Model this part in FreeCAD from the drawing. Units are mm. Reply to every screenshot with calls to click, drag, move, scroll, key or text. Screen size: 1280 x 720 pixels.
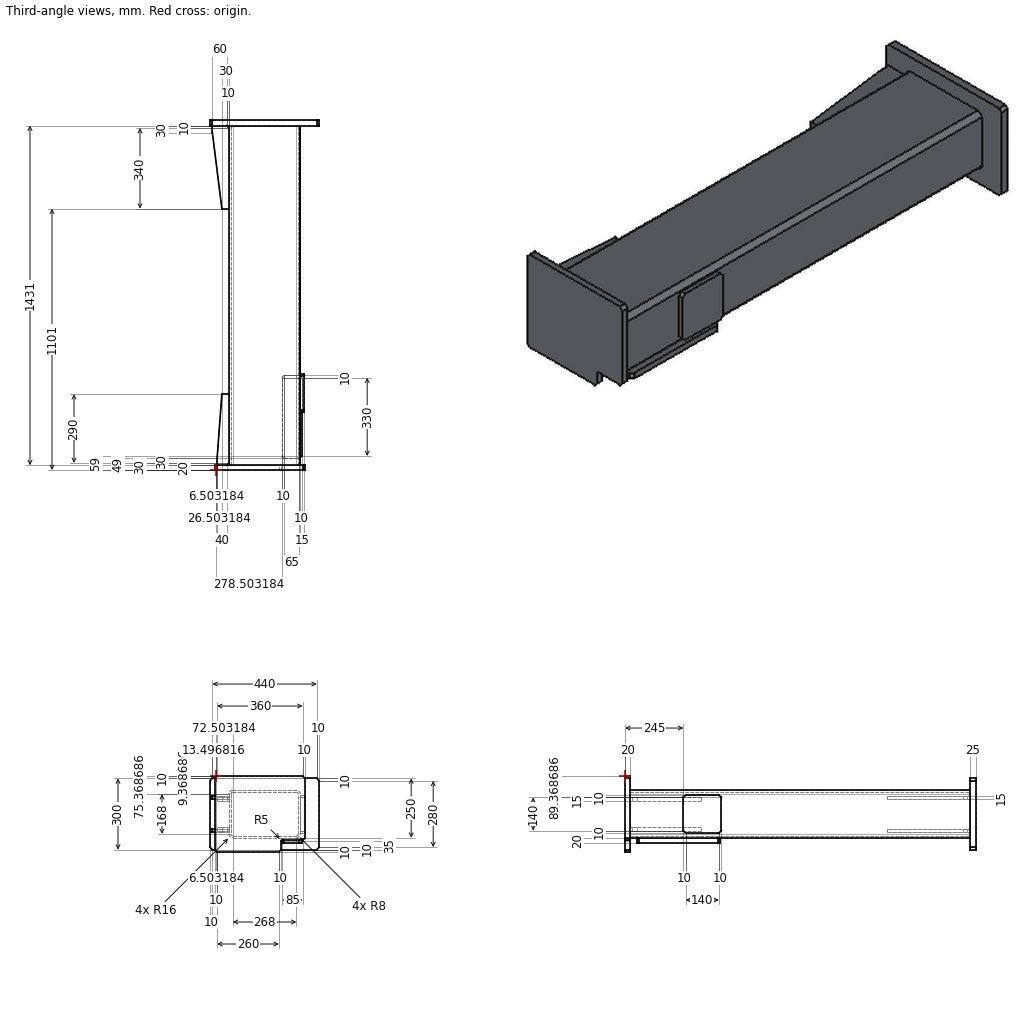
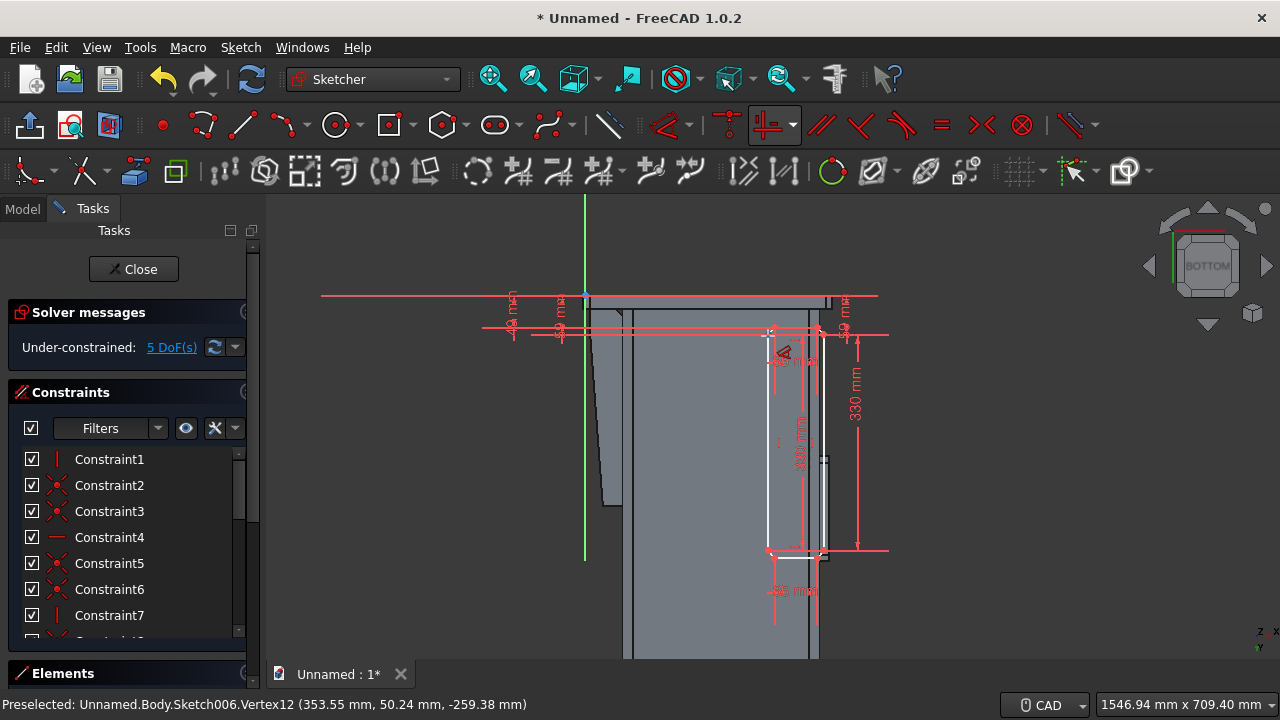
scroll(771, 554, up, 10)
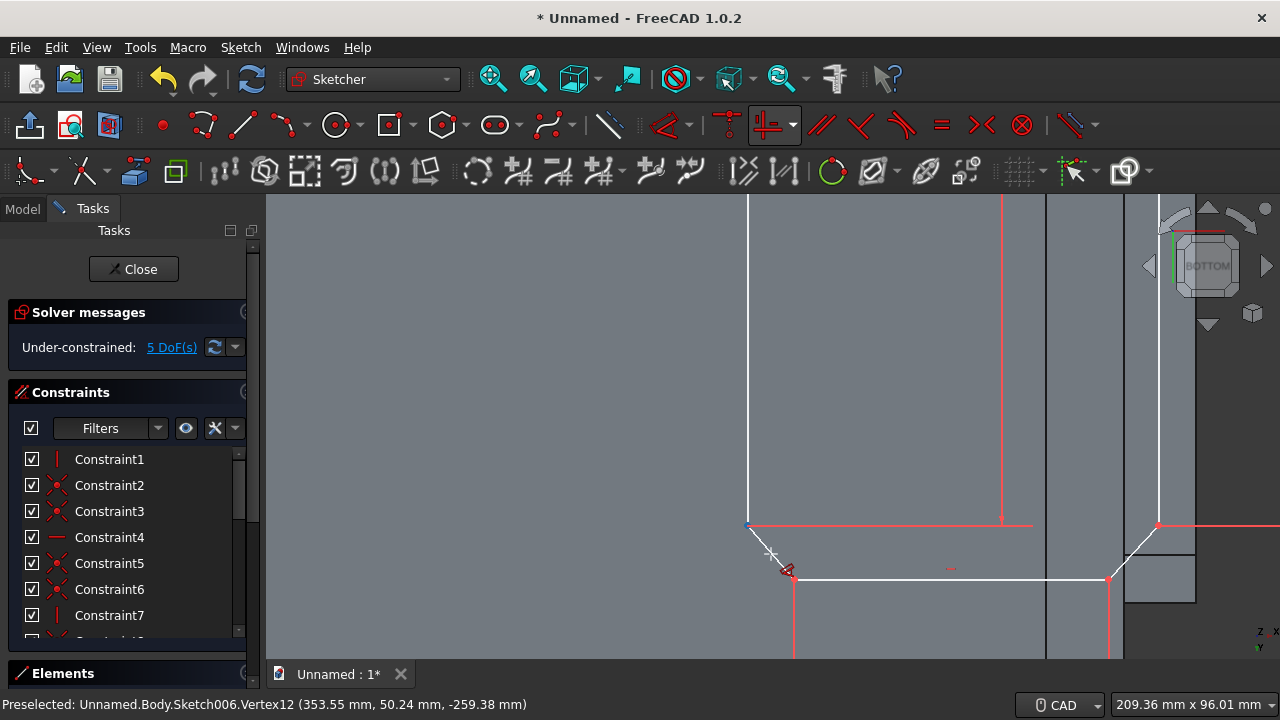
click(771, 553)
click(771, 614)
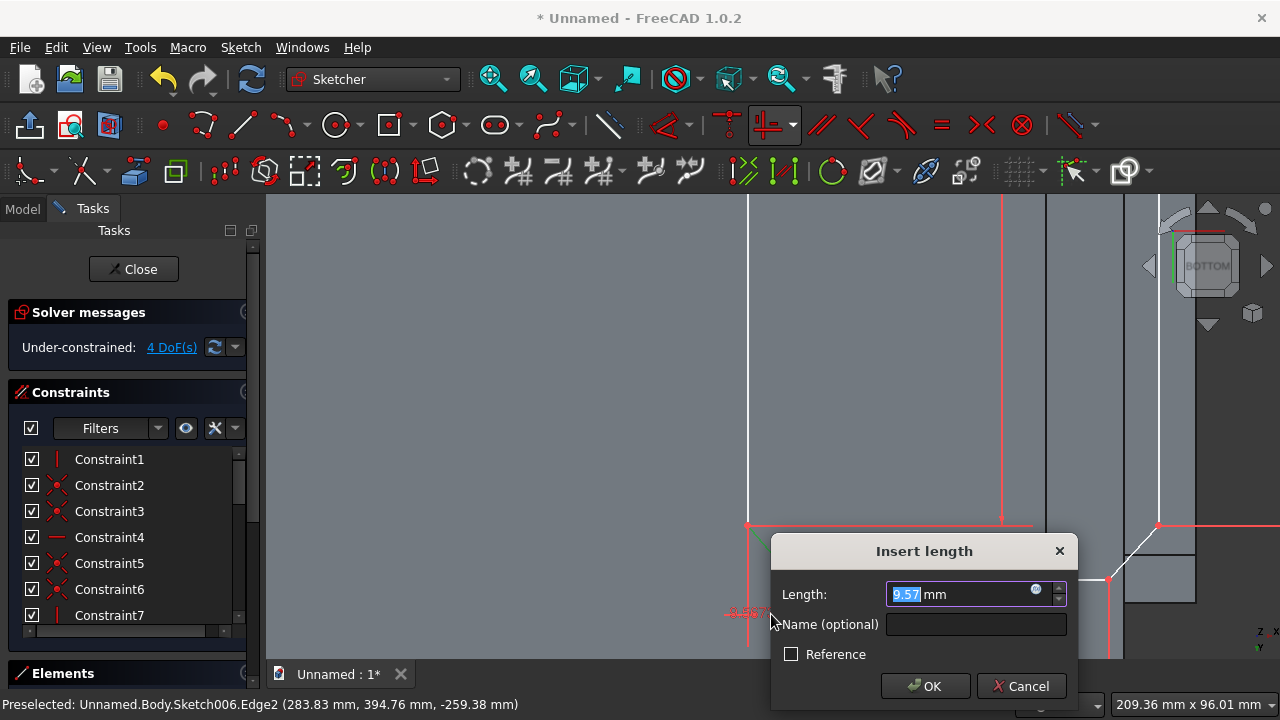
text(10)
key(Return)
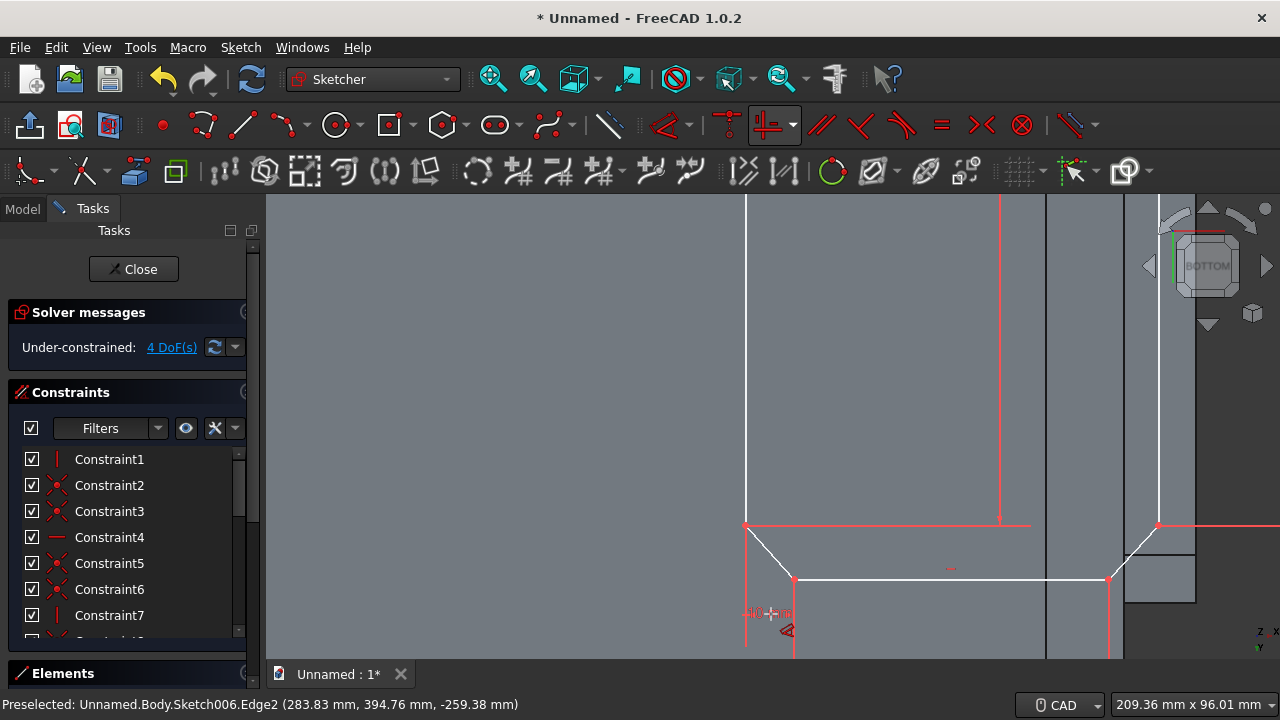
click(760, 542)
click(828, 553)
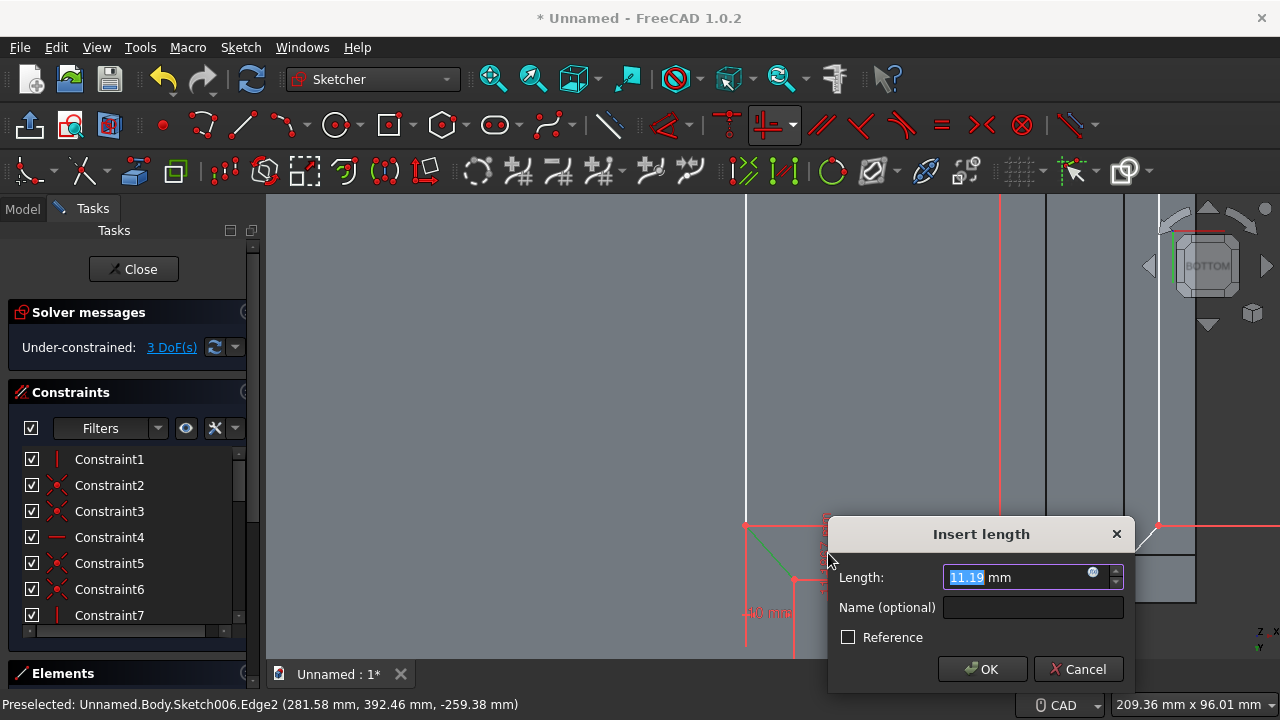
text(10)
key(Return)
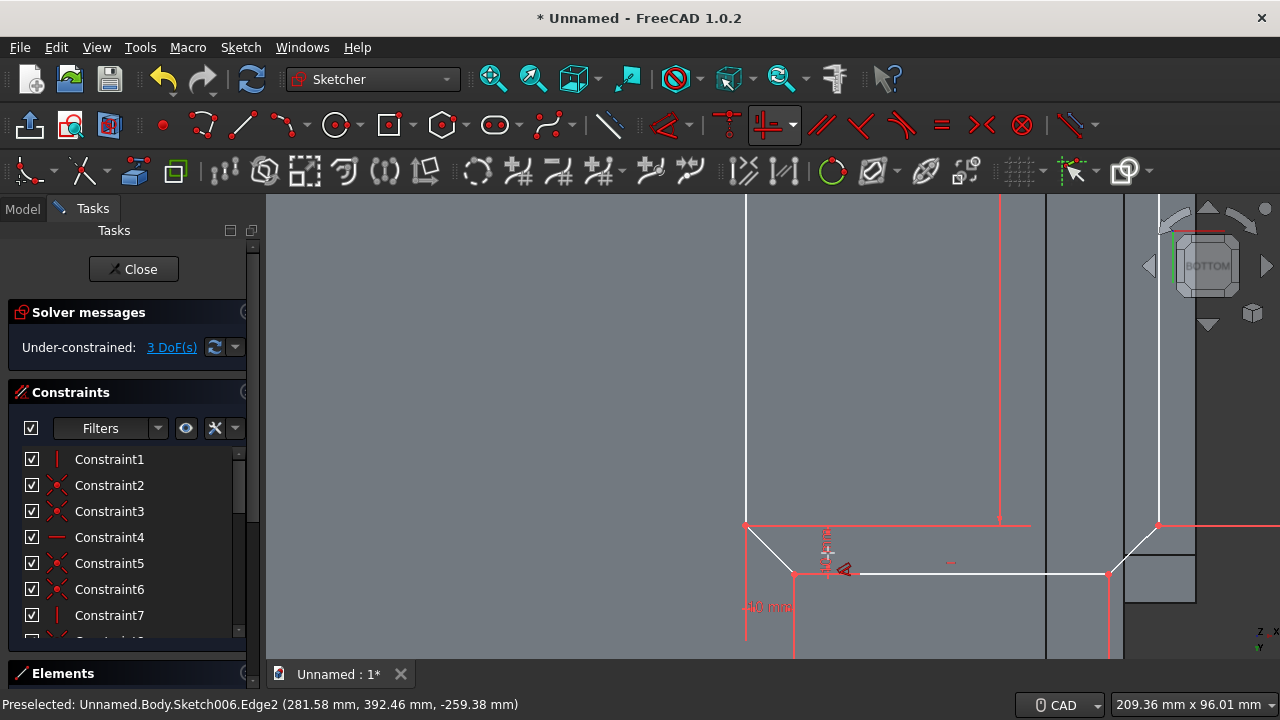
scroll(771, 555, down, 10)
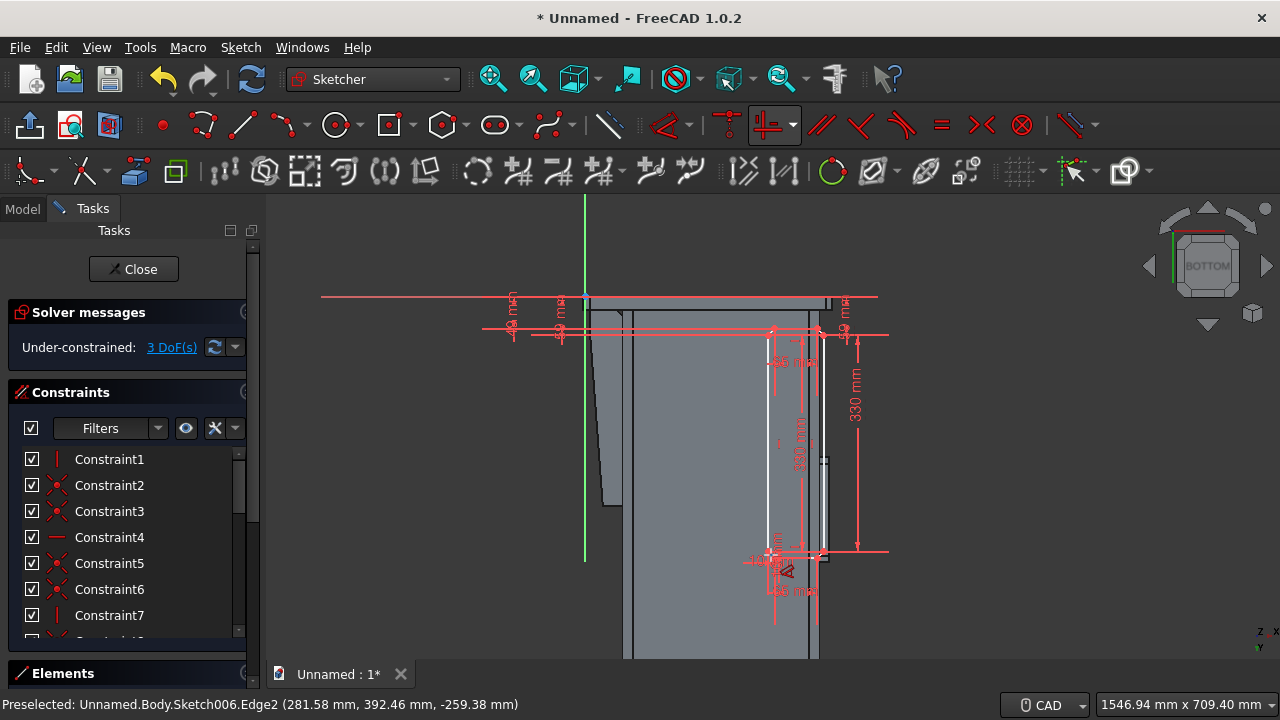
scroll(819, 556, up, 10)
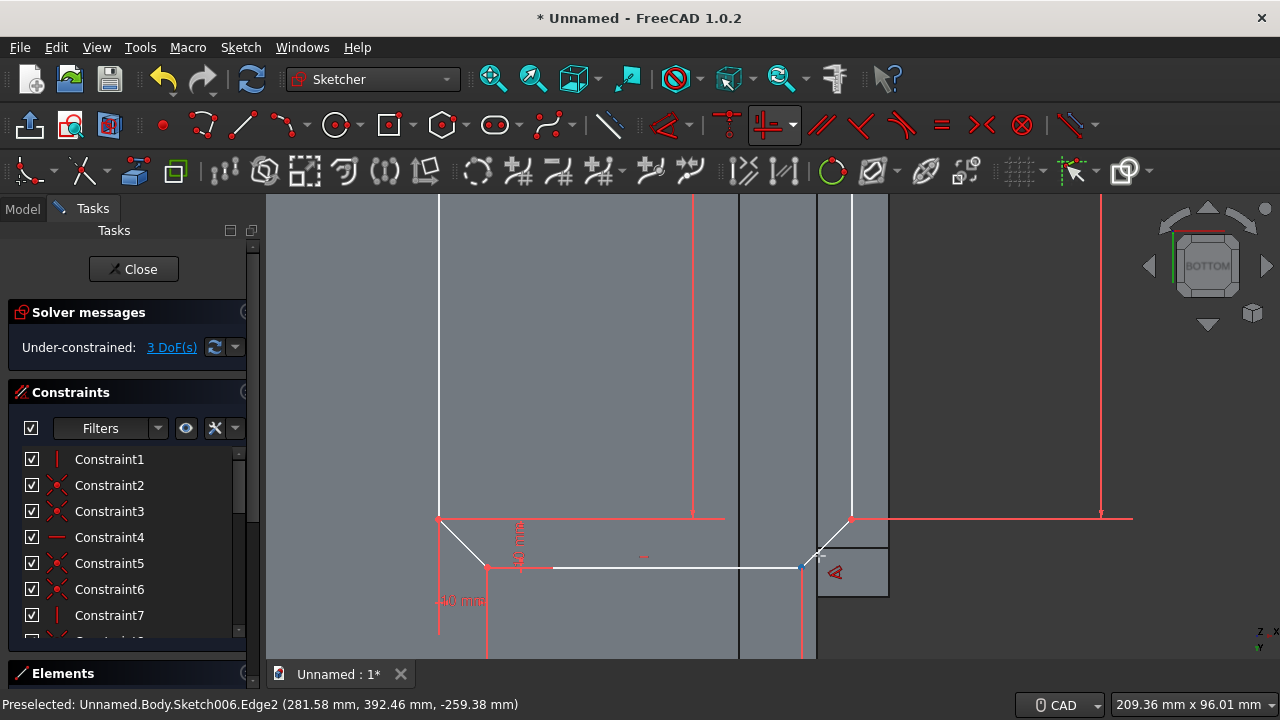
click(817, 553)
click(827, 602)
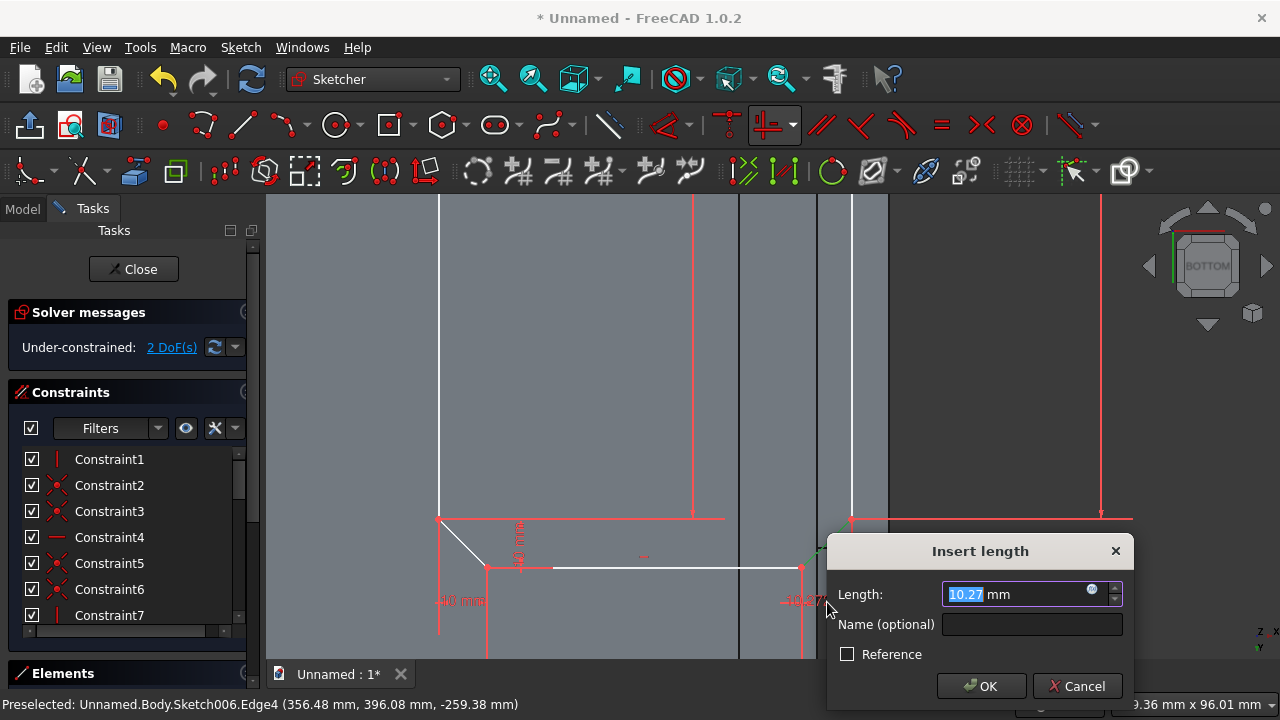
text(10)
key(Return)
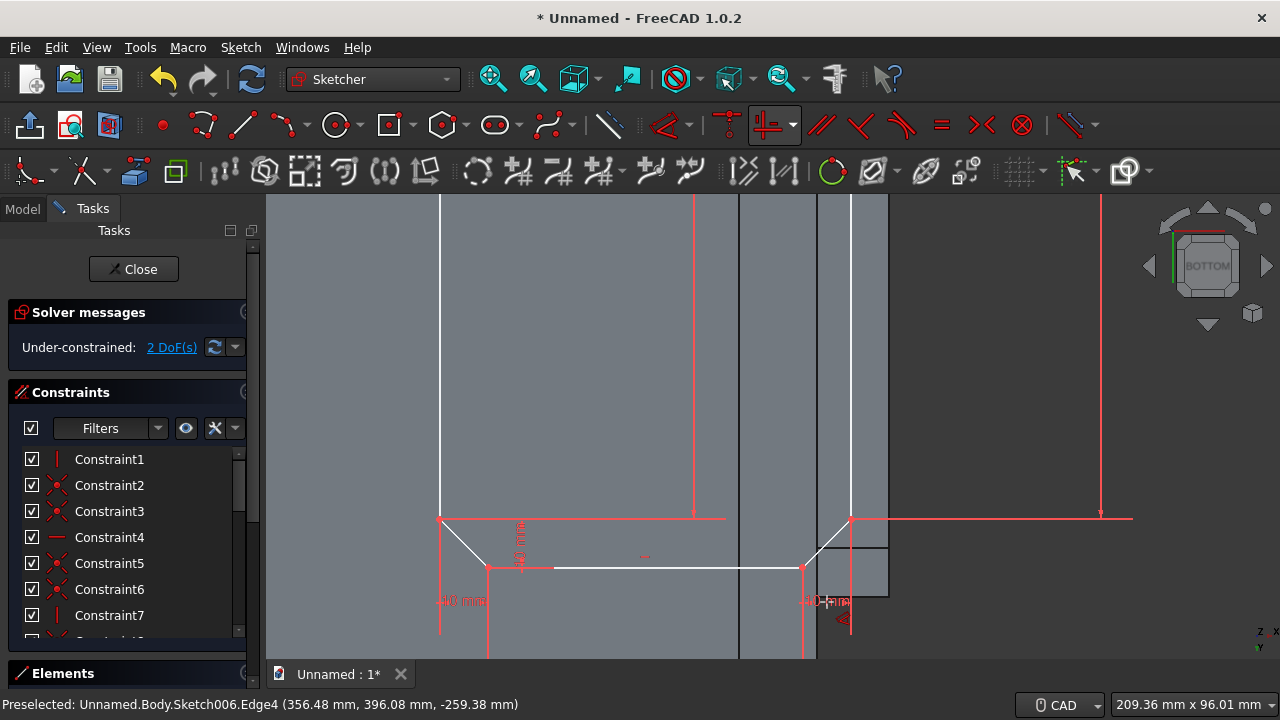
scroll(819, 556, down, 10)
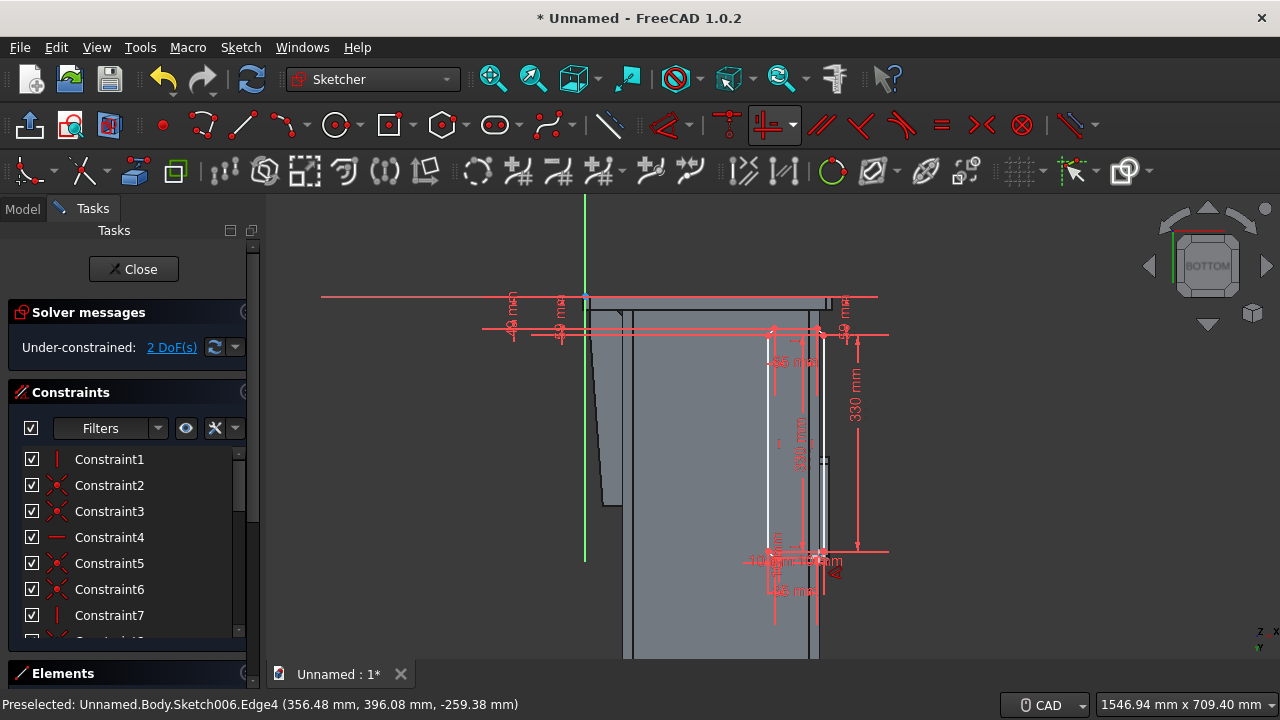
scroll(822, 333, up, 10)